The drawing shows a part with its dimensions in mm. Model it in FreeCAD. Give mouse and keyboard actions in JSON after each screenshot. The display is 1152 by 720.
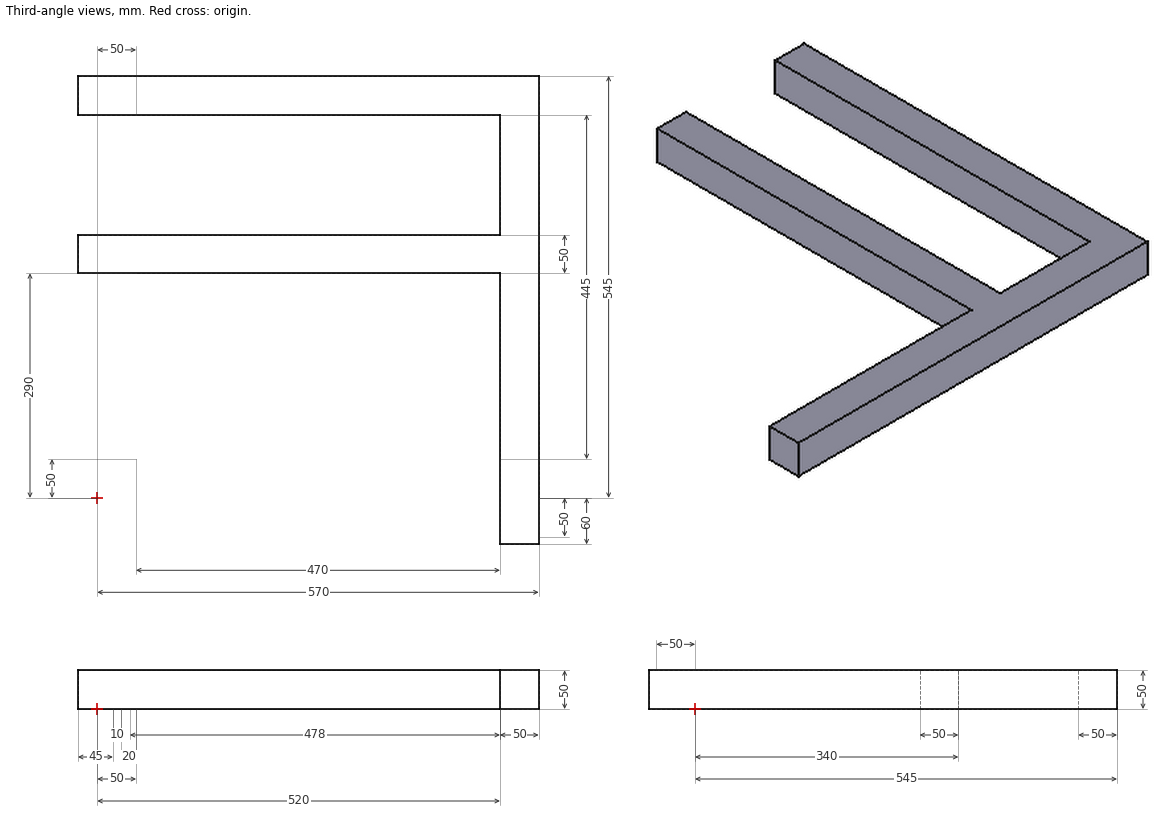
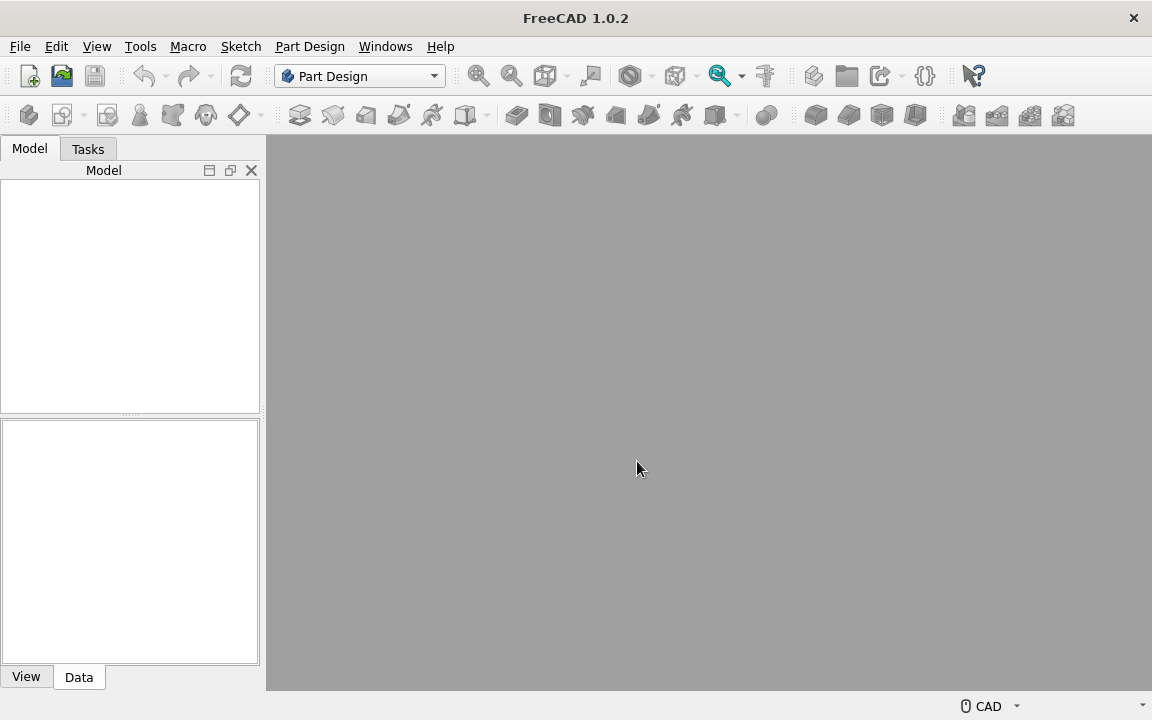
{"action": "left_click", "coordinate": [29, 76]}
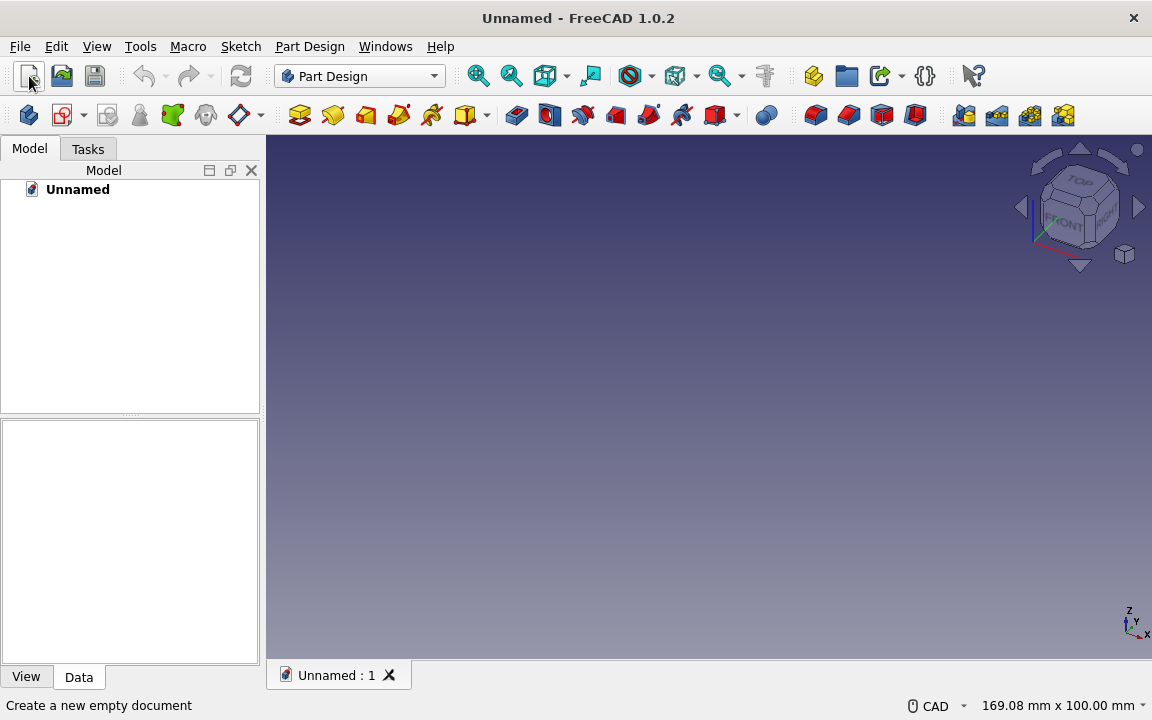
{"action": "left_click", "coordinate": [62, 116]}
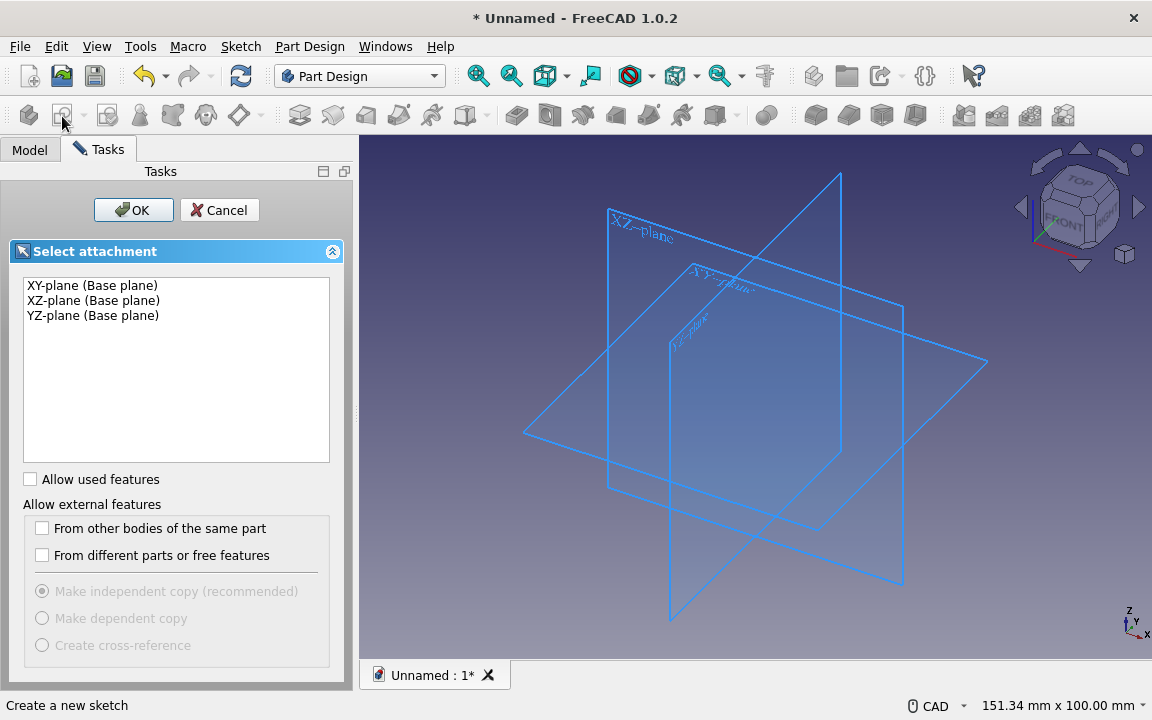
{"action": "left_click", "coordinate": [84, 286]}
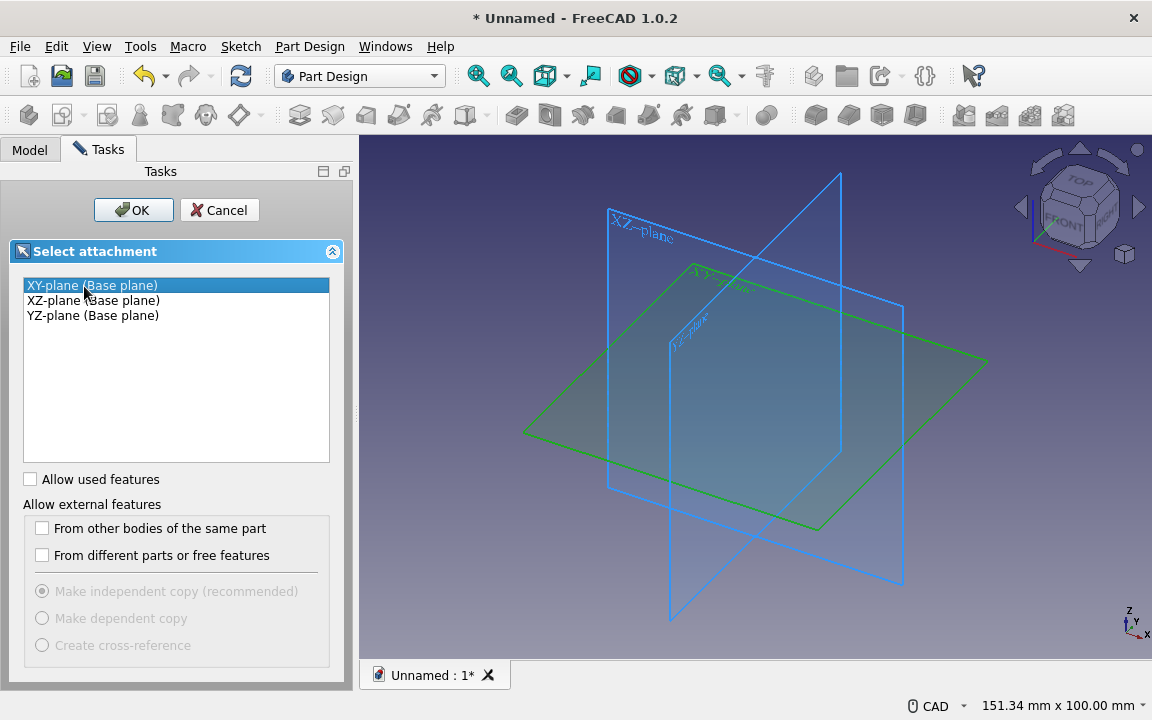
{"action": "left_click", "coordinate": [134, 210]}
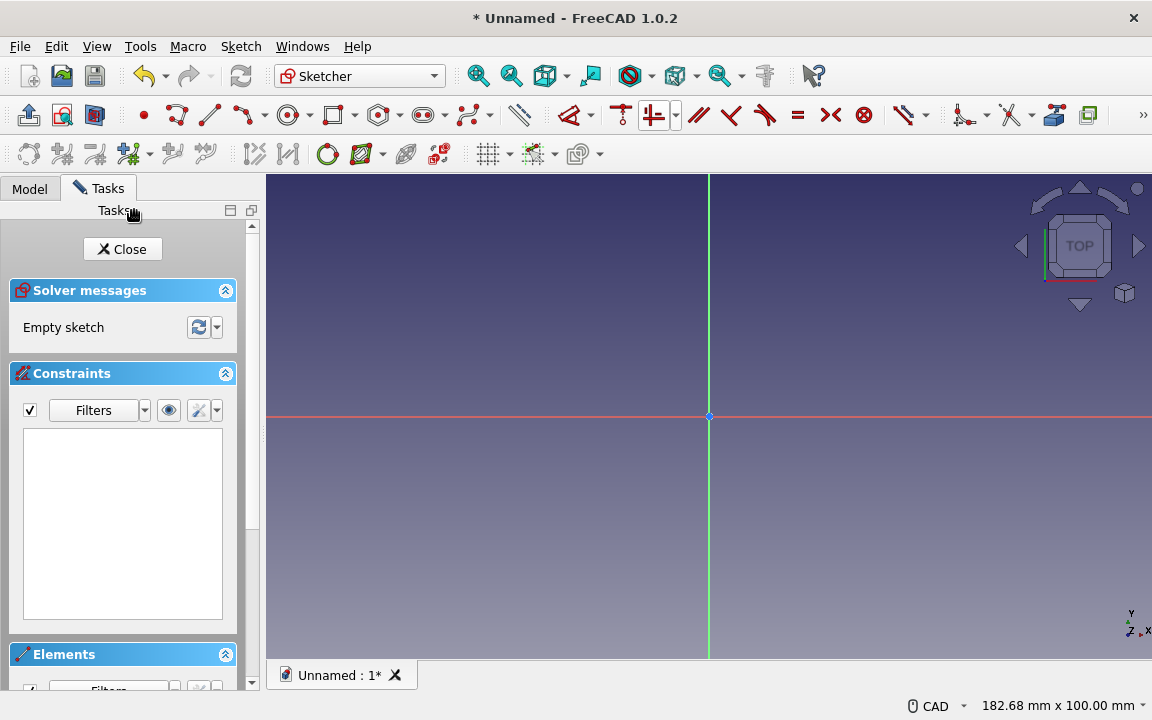
{"action": "scroll", "coordinate": [460, 581], "scroll_direction": "down", "scroll_amount": 11}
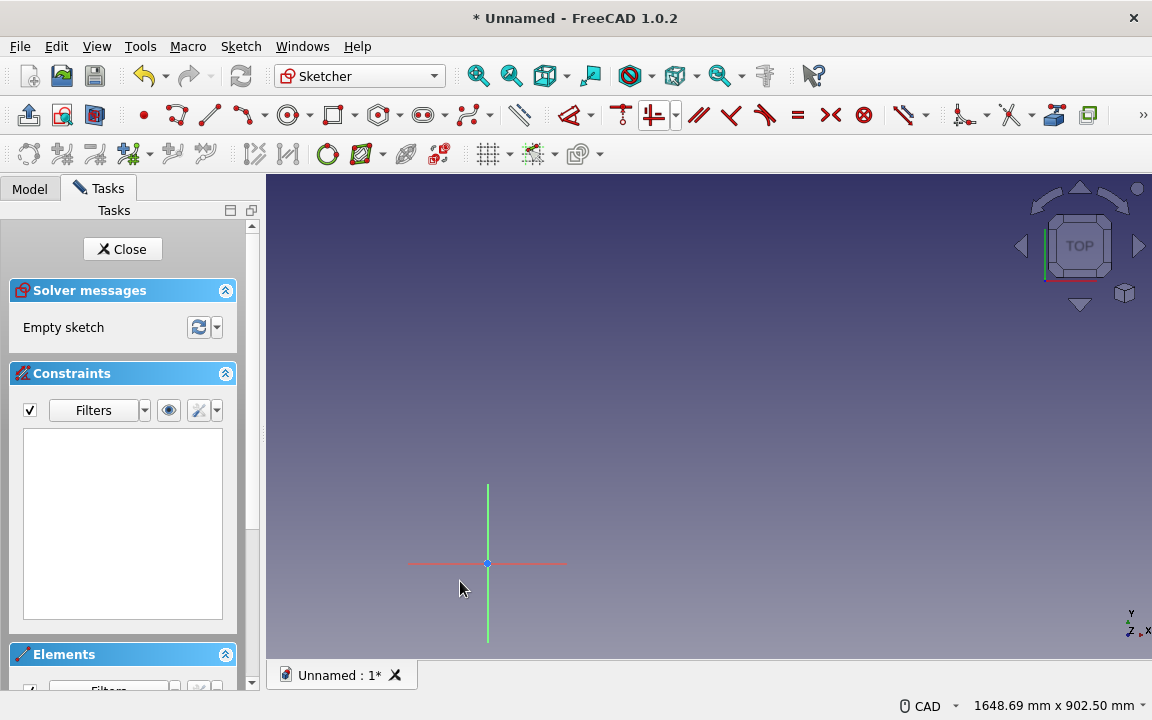
{"action": "key", "text": "g r"}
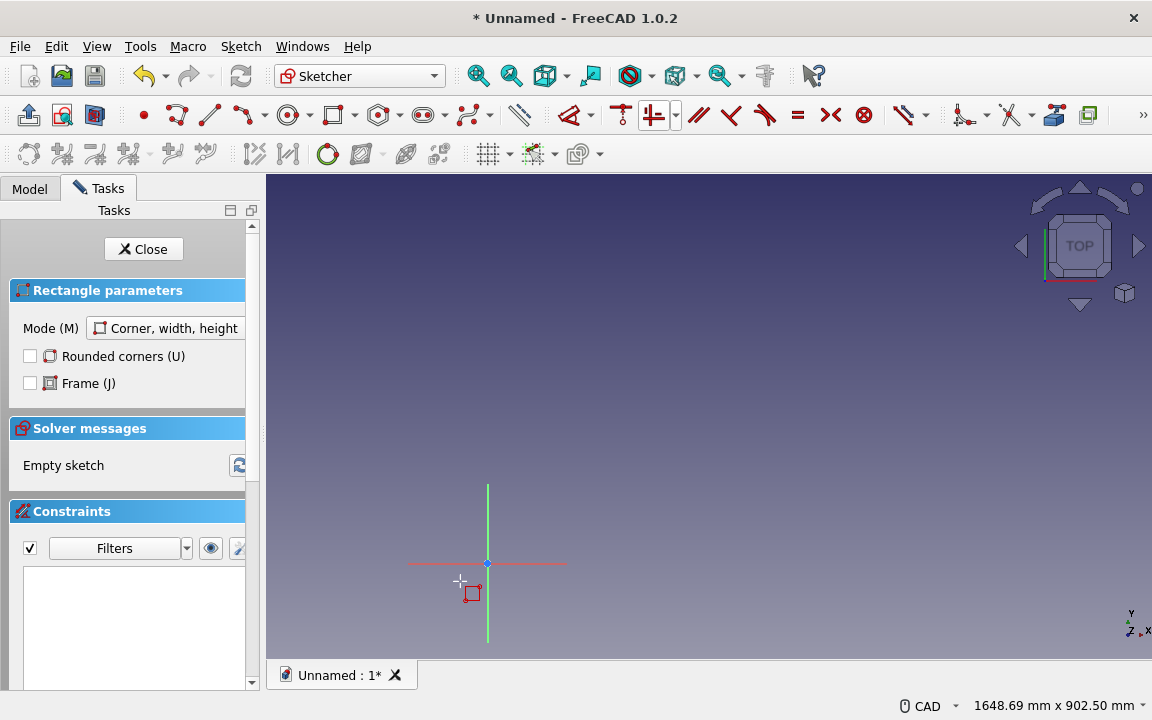
{"action": "left_click", "coordinate": [488, 564]}
{"action": "mouse_move", "coordinate": [794, 271]}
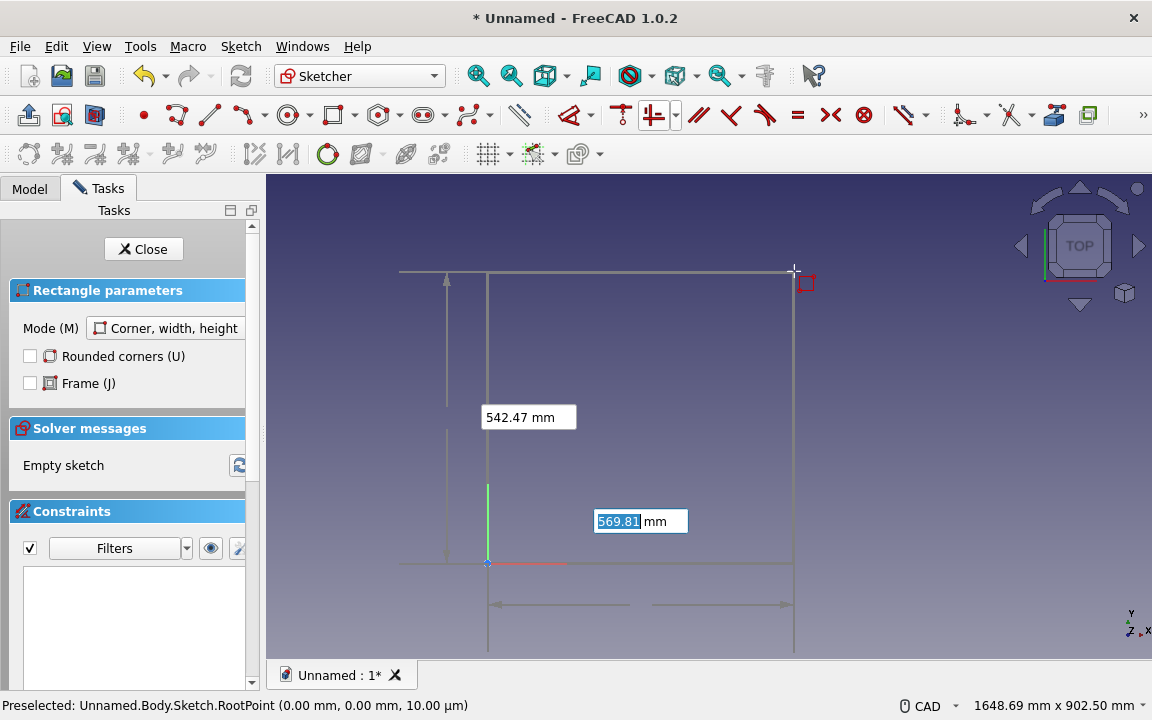
{"action": "type", "text": "570"}
{"action": "key", "text": "Tab"}
{"action": "type", "text": "545"}
{"action": "key", "text": "Return"}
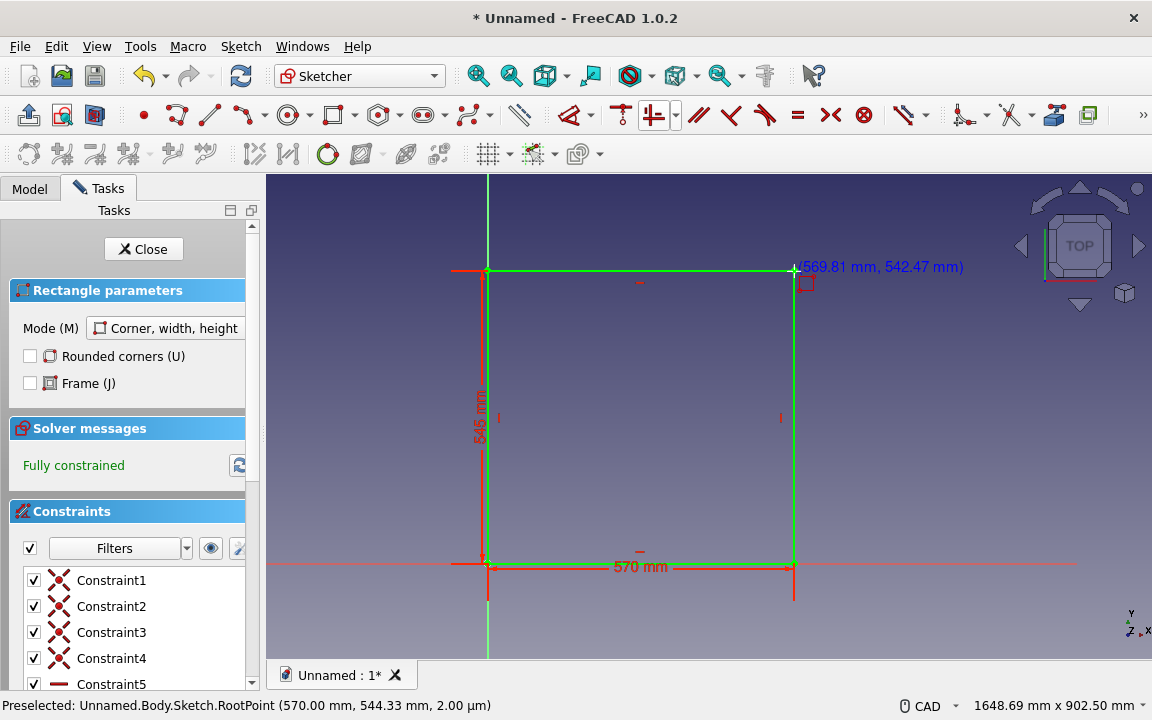
{"action": "left_click", "coordinate": [515, 298]}
{"action": "mouse_move", "coordinate": [767, 537]}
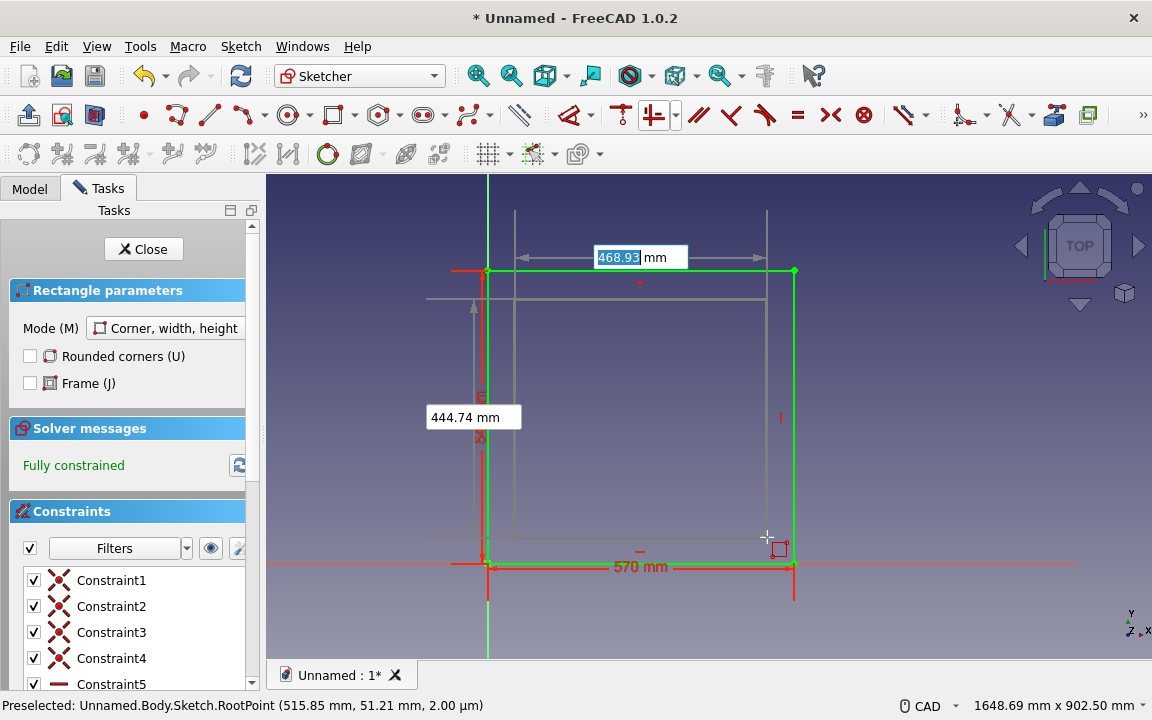
{"action": "type", "text": "470"}
{"action": "key", "text": "Tab"}
{"action": "type", "text": "445"}
{"action": "key", "text": "Return"}
{"action": "key", "text": "Escape"}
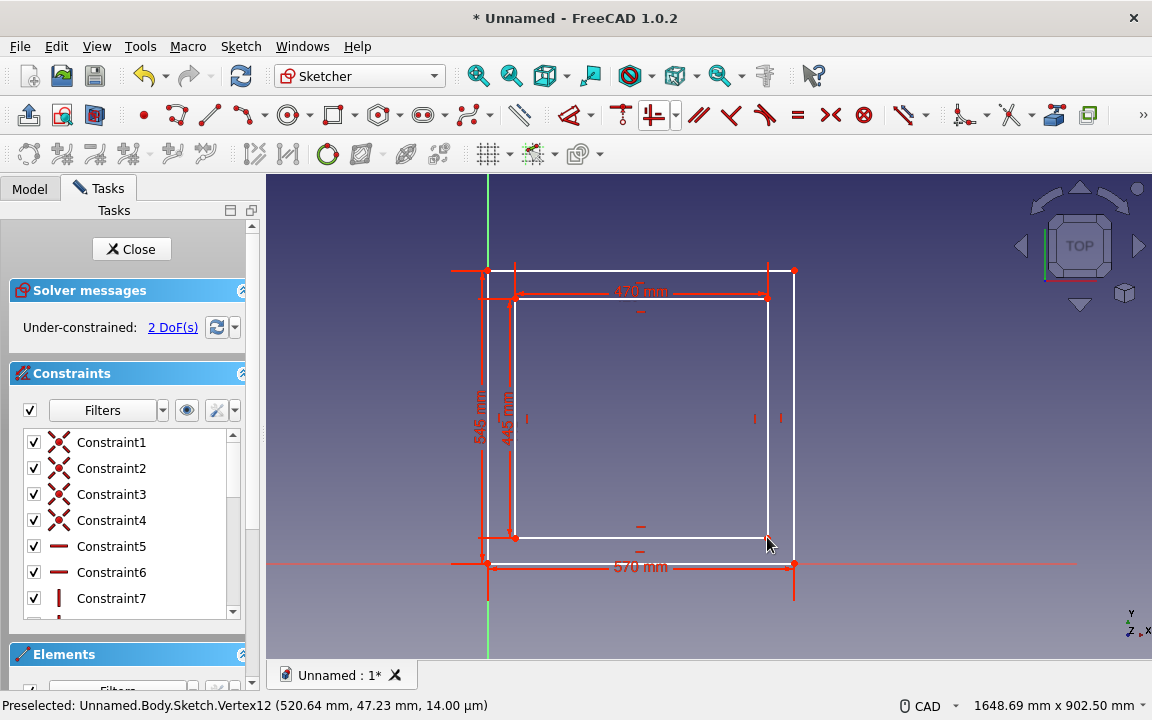
{"action": "scroll", "coordinate": [515, 299], "scroll_direction": "up", "scroll_amount": 2}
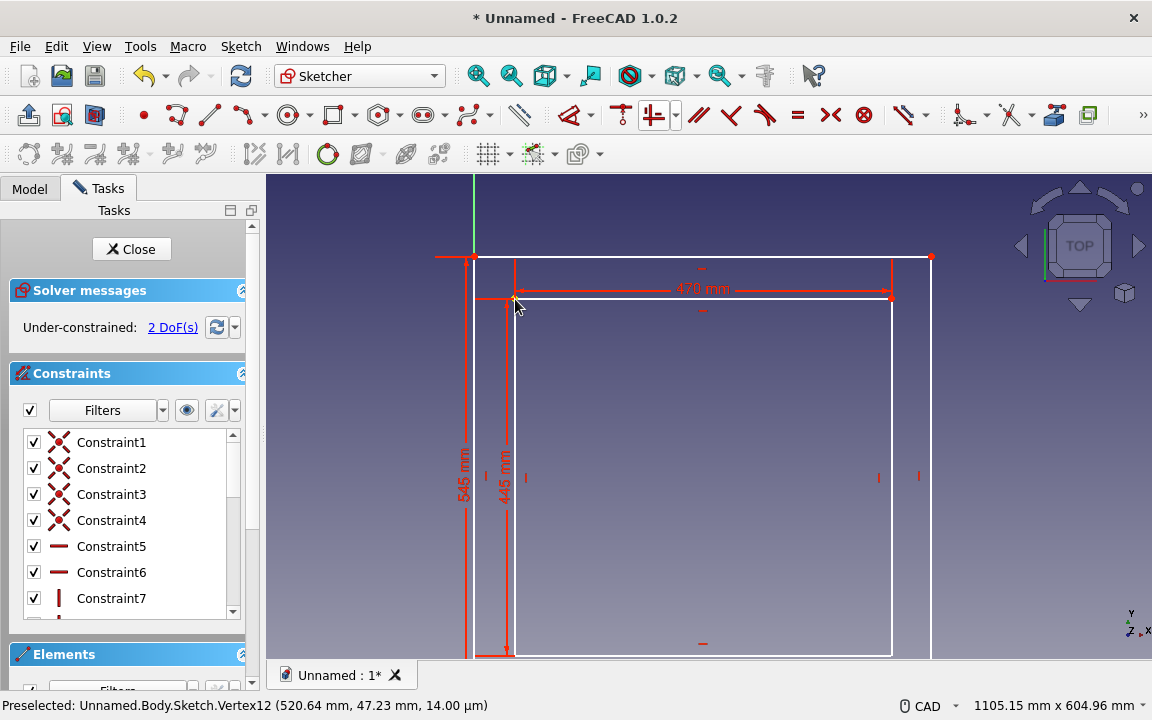
{"action": "left_click", "coordinate": [515, 299]}